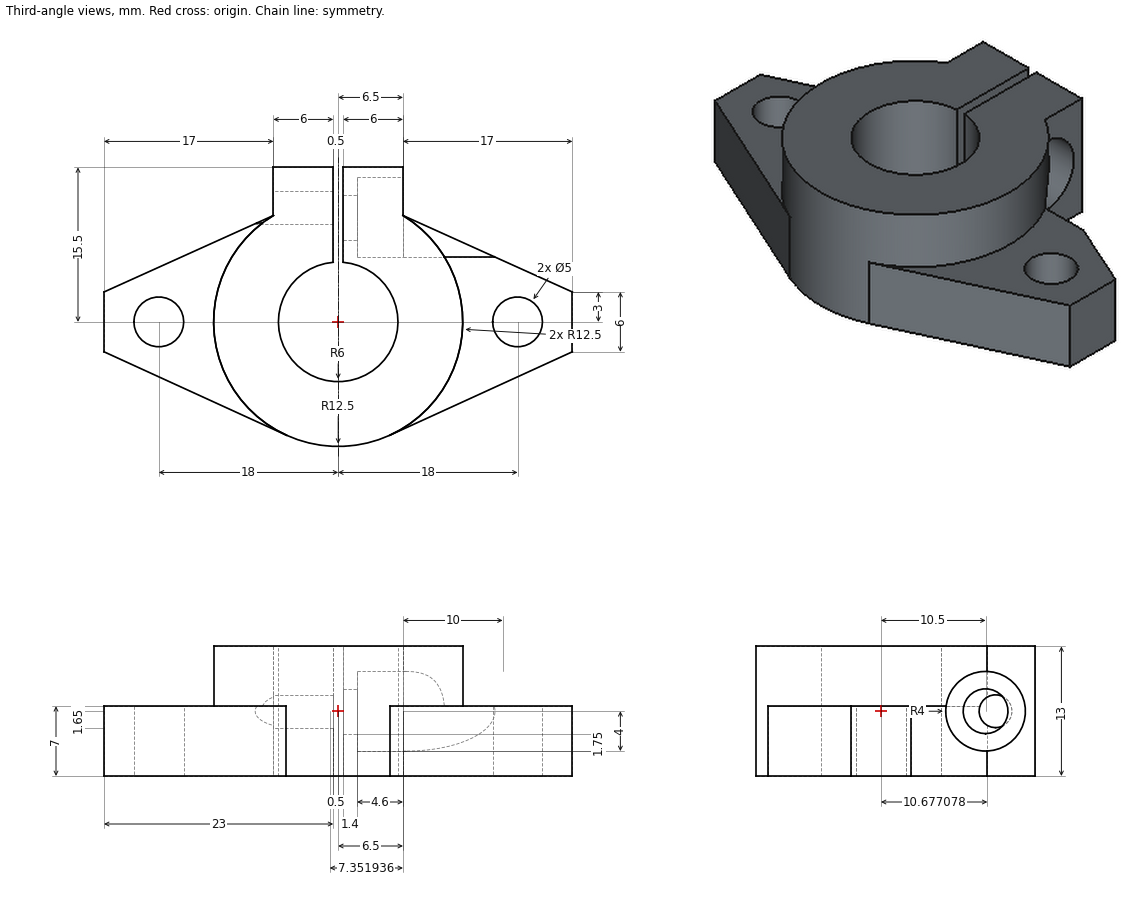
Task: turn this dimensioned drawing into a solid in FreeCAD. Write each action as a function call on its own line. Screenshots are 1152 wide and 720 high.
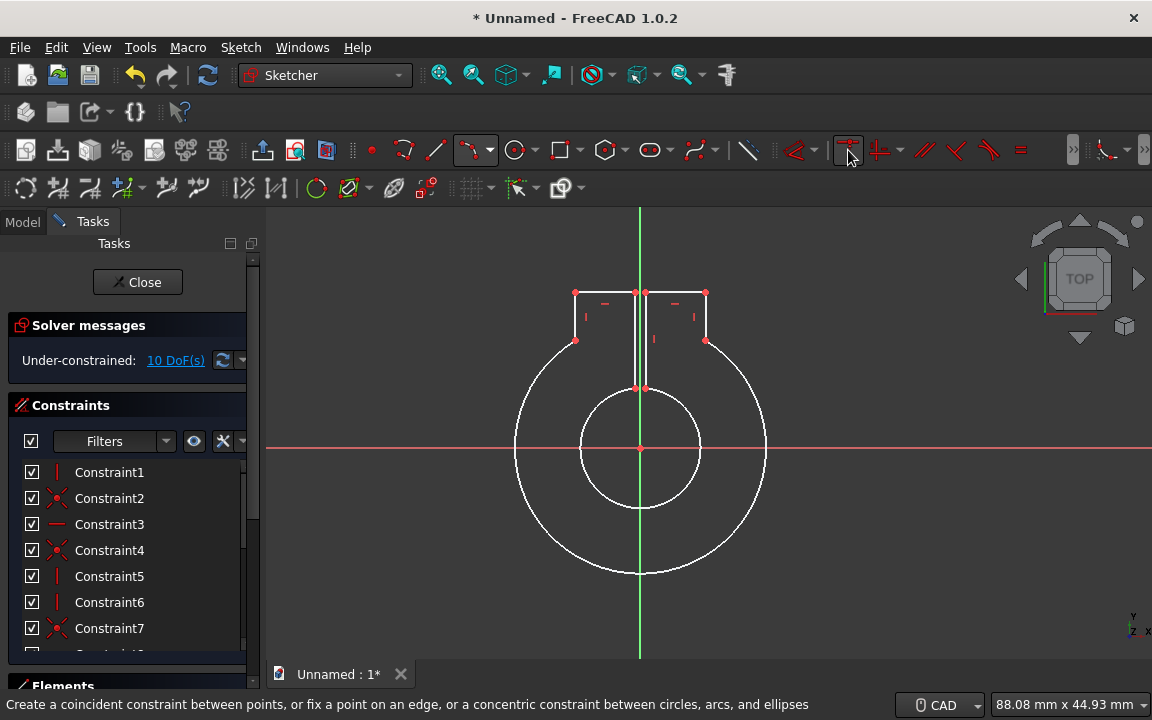
drag(630, 438, 650, 458)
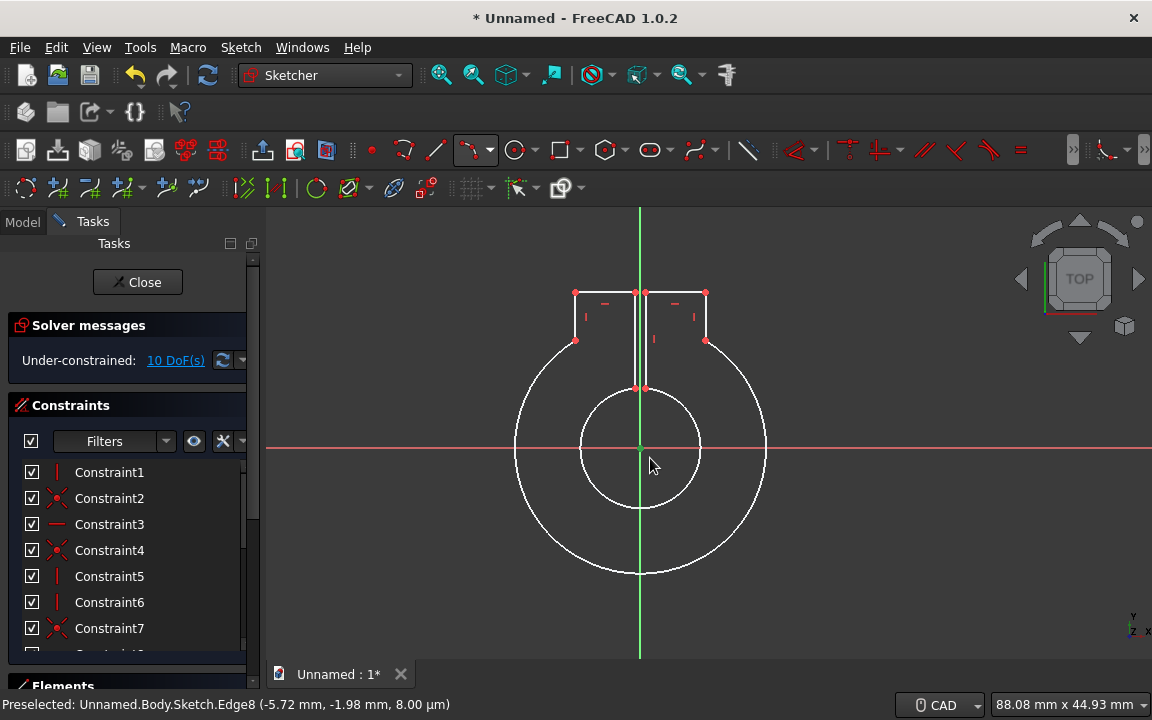
click(848, 150)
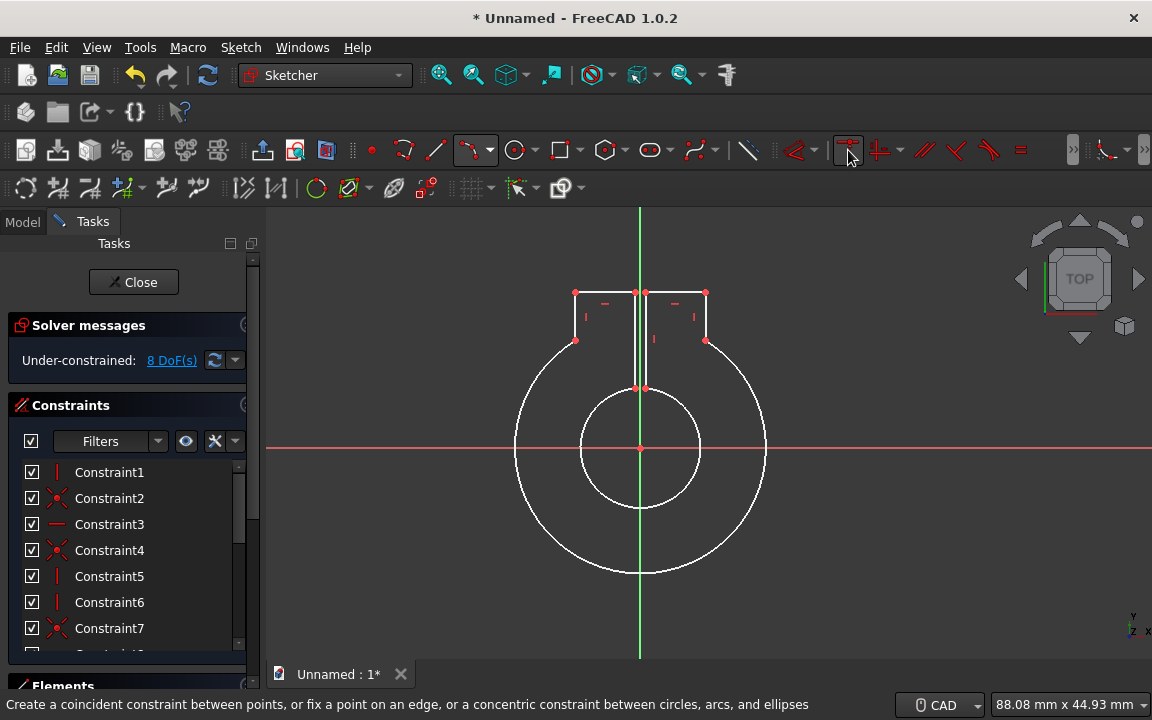
click(575, 292)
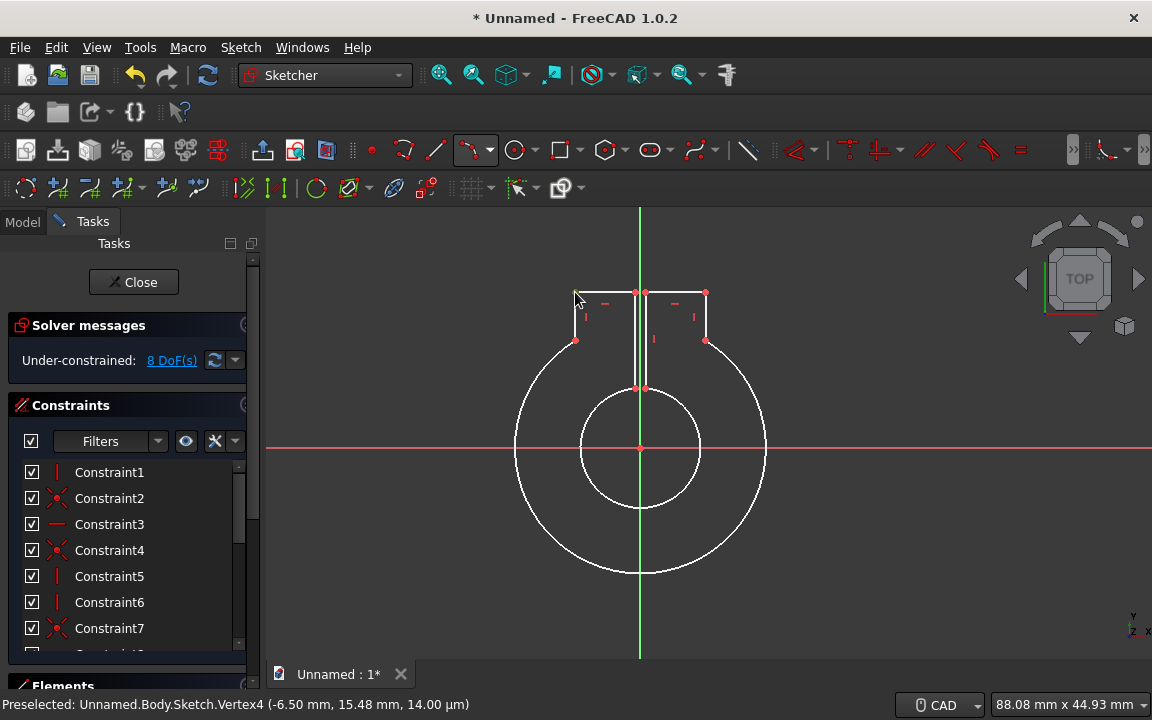
click(706, 292)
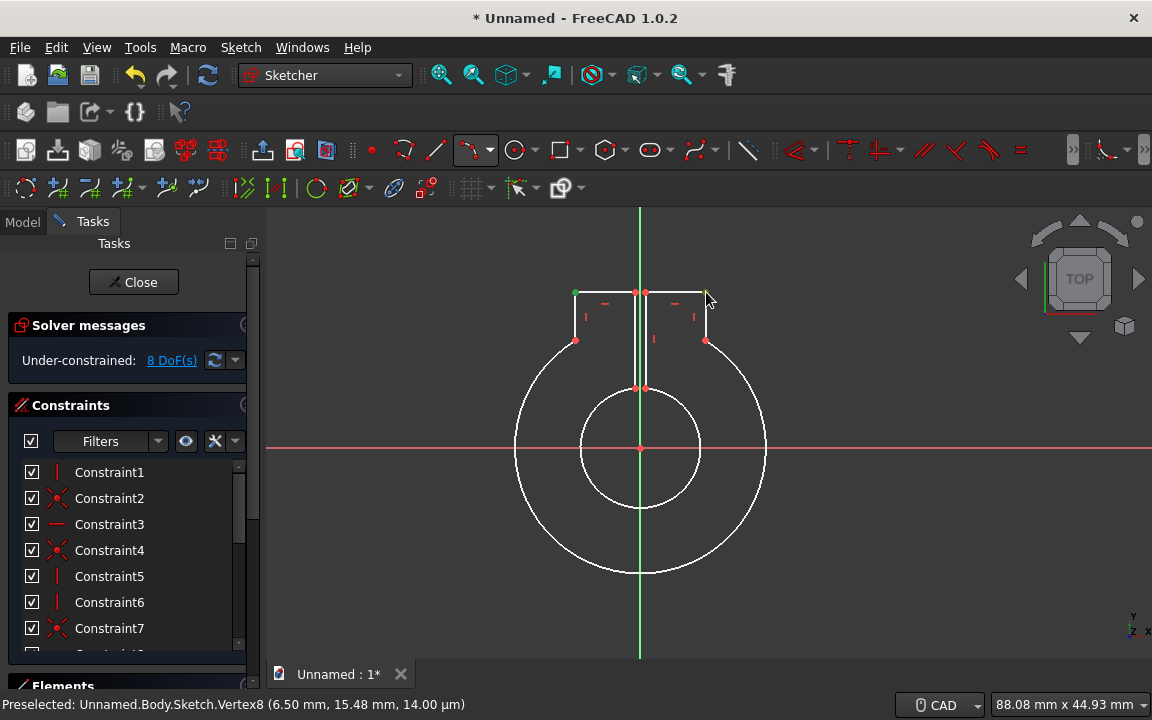
click(640, 263)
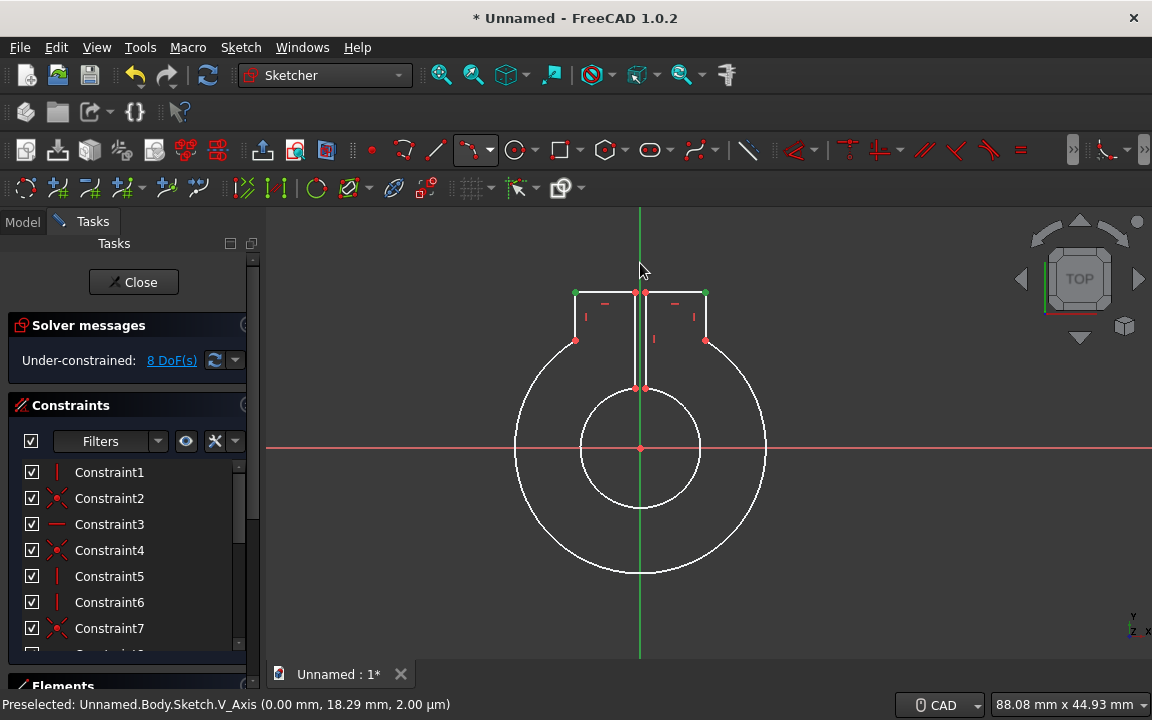
key(s)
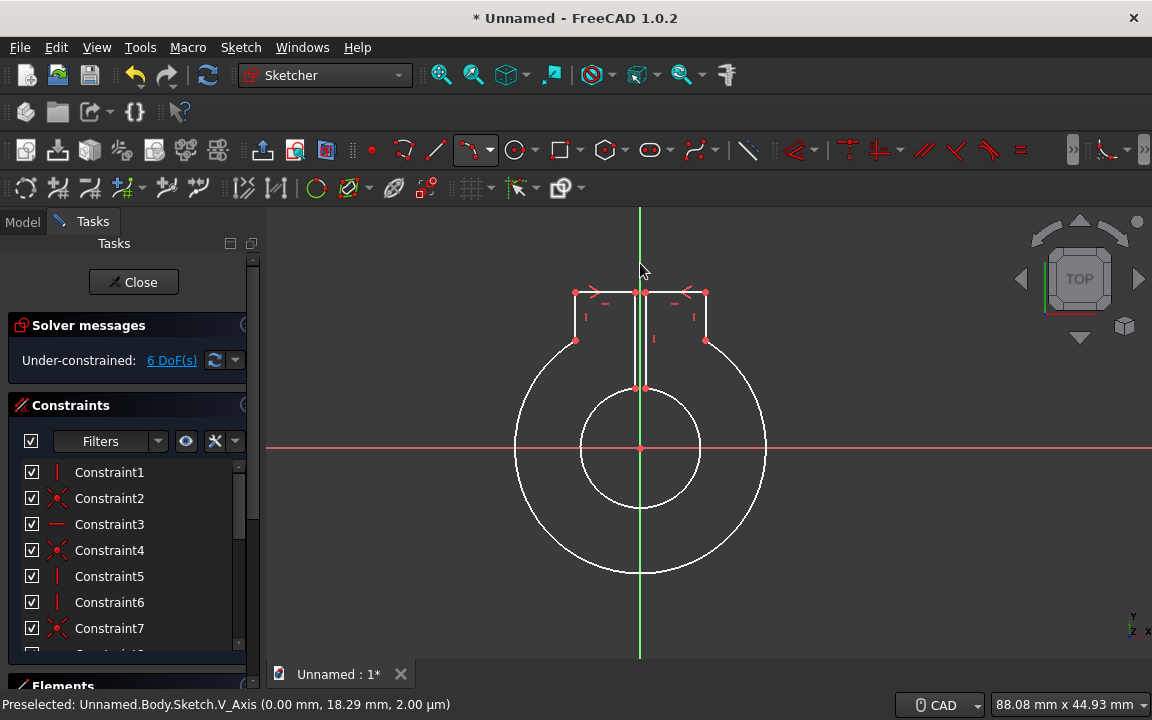
click(794, 150)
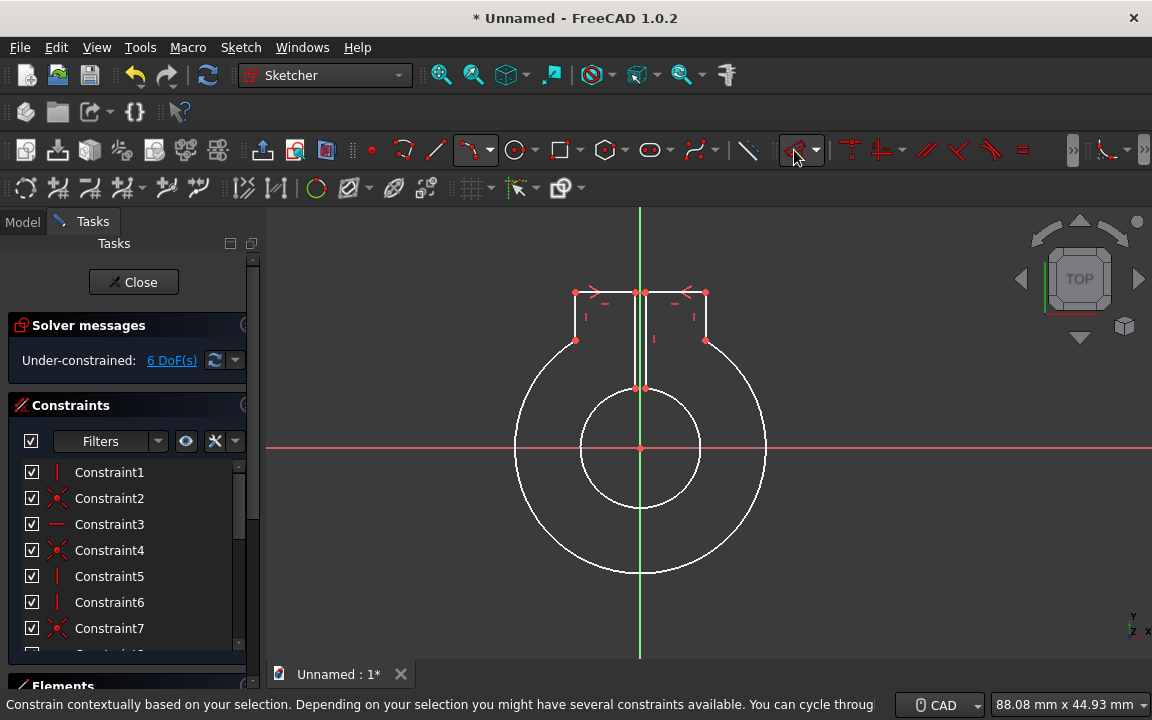
click(532, 512)
click(504, 528)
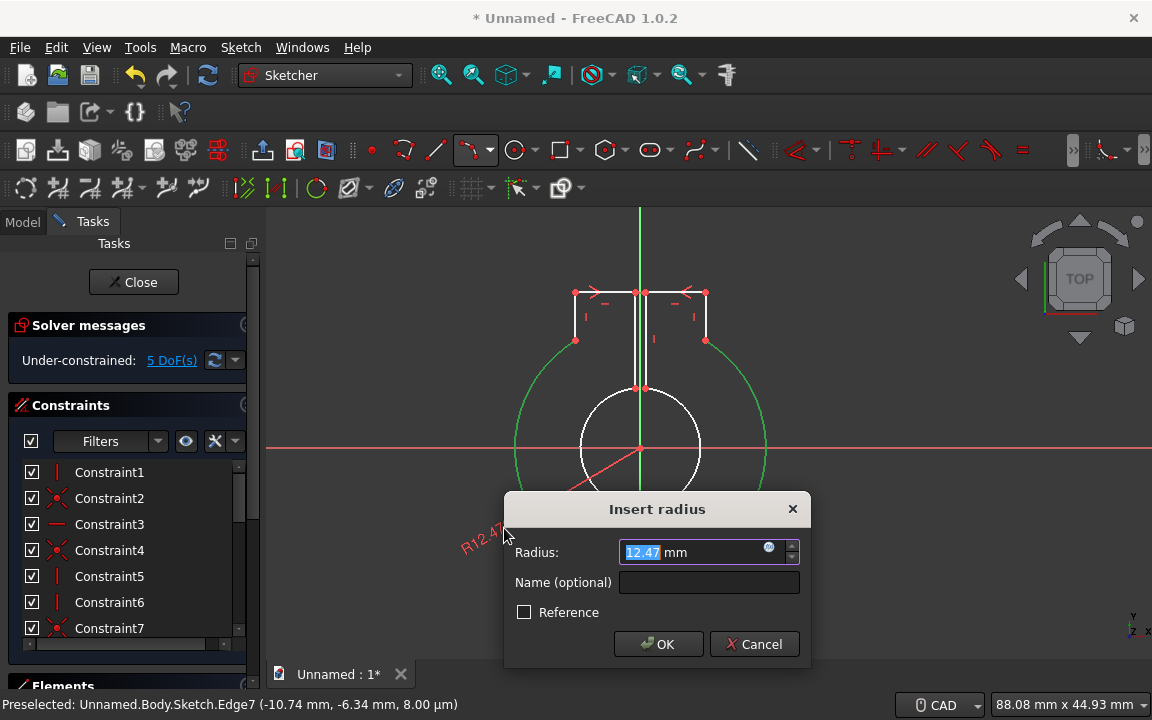
text(12.5)
key(Return)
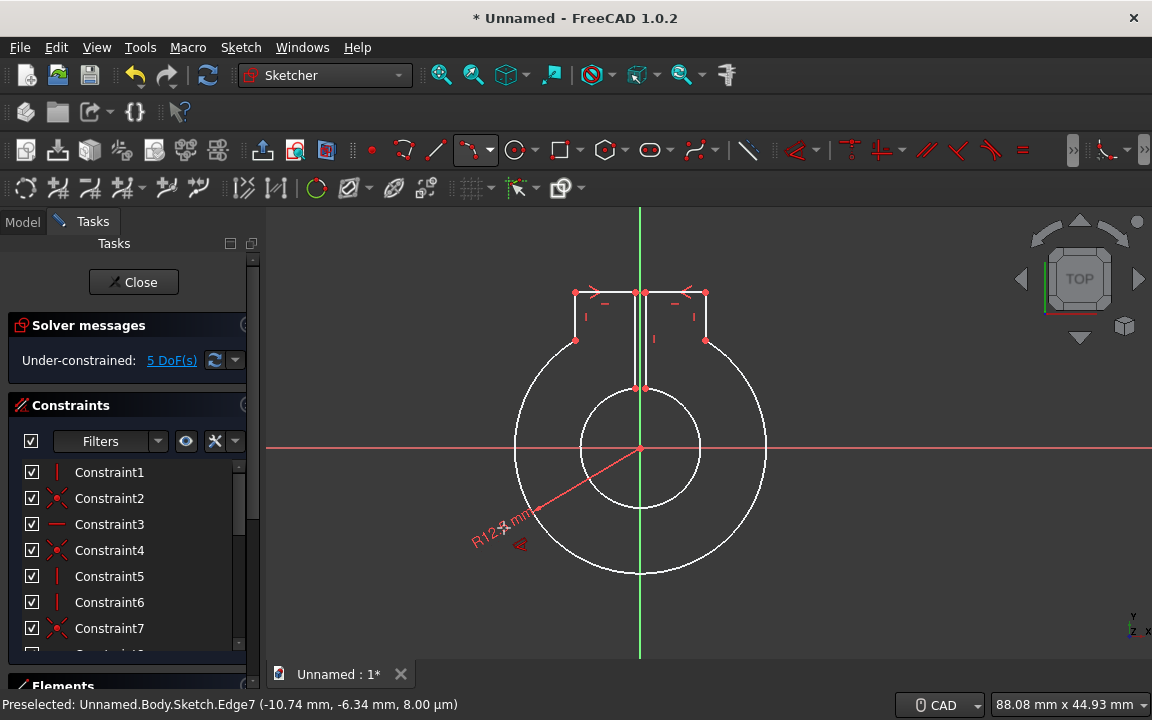
click(584, 468)
click(554, 479)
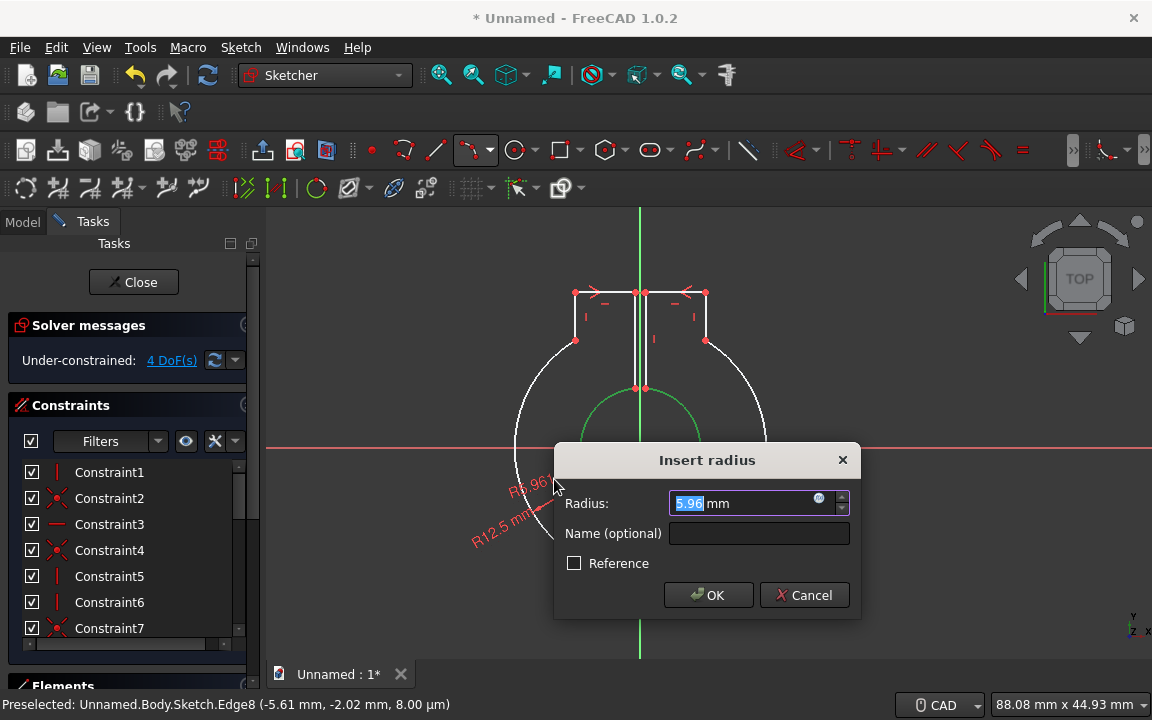
text(6)
key(Return)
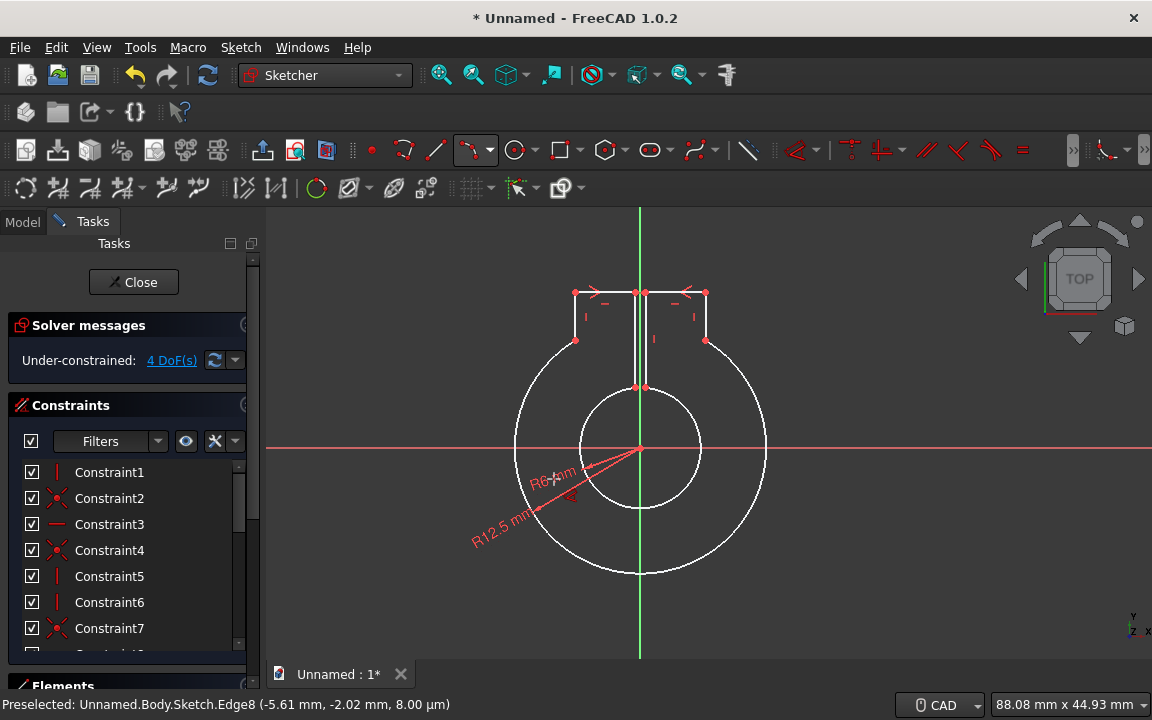
click(617, 292)
click(605, 258)